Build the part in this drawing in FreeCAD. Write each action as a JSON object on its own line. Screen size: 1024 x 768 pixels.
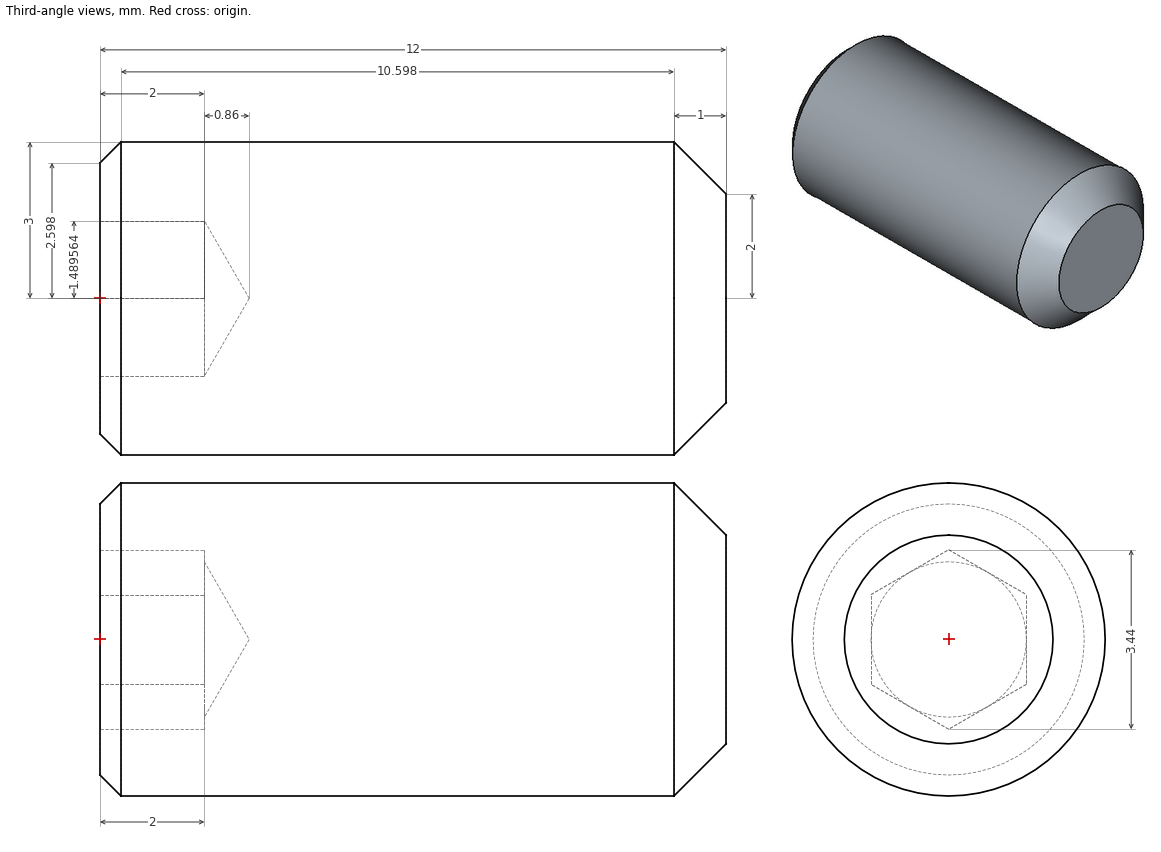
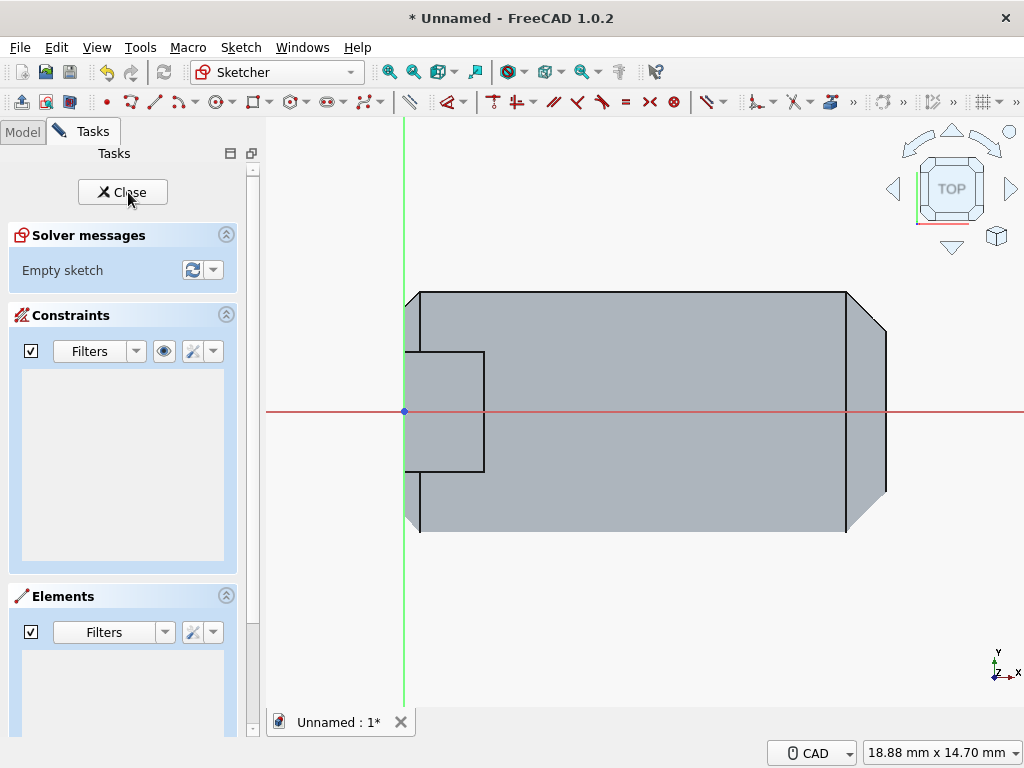
{"action": "scroll", "coordinate": [412, 369], "scroll_direction": "up", "scroll_amount": 6}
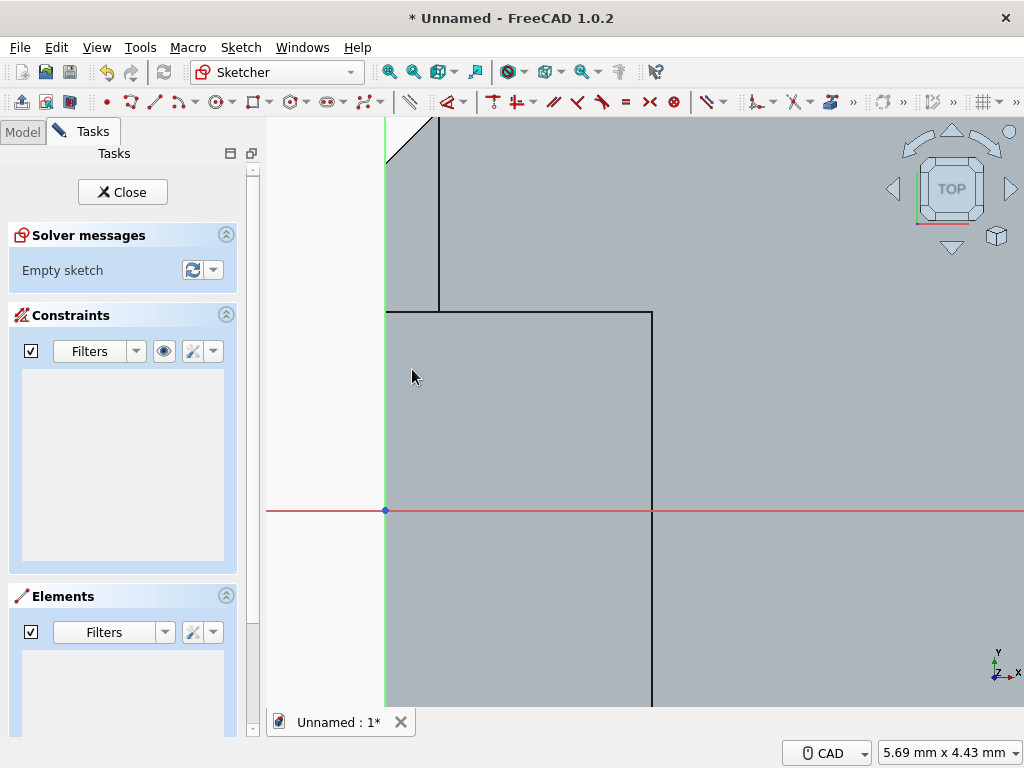
{"action": "key", "text": "g m"}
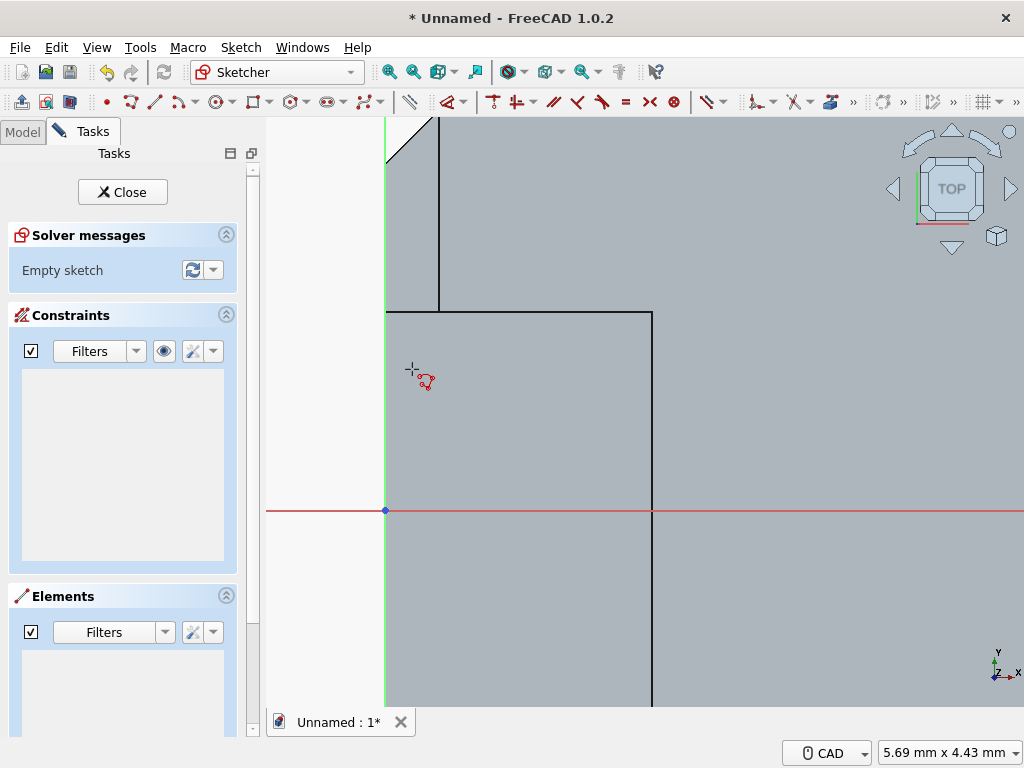
{"action": "left_click", "coordinate": [652, 511]}
{"action": "left_click", "coordinate": [767, 502]}
{"action": "left_click", "coordinate": [652, 312]}
{"action": "left_click", "coordinate": [652, 511]}
{"action": "key", "text": "Escape"}
{"action": "key", "text": "Escape"}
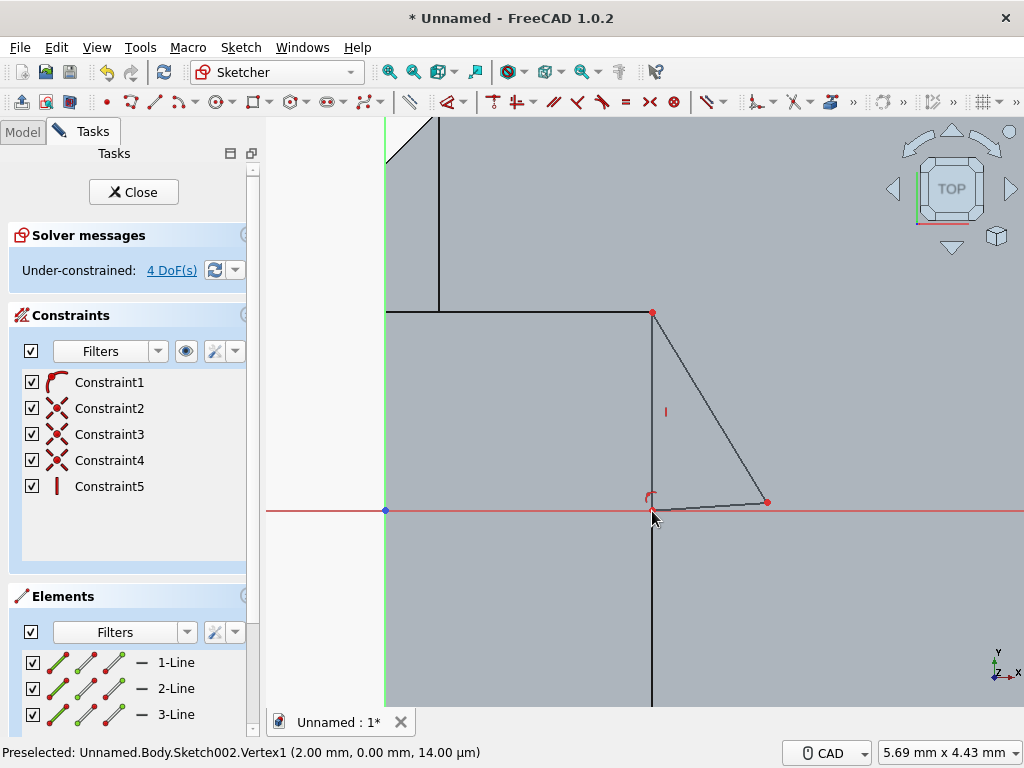
{"action": "left_click", "coordinate": [686, 508]}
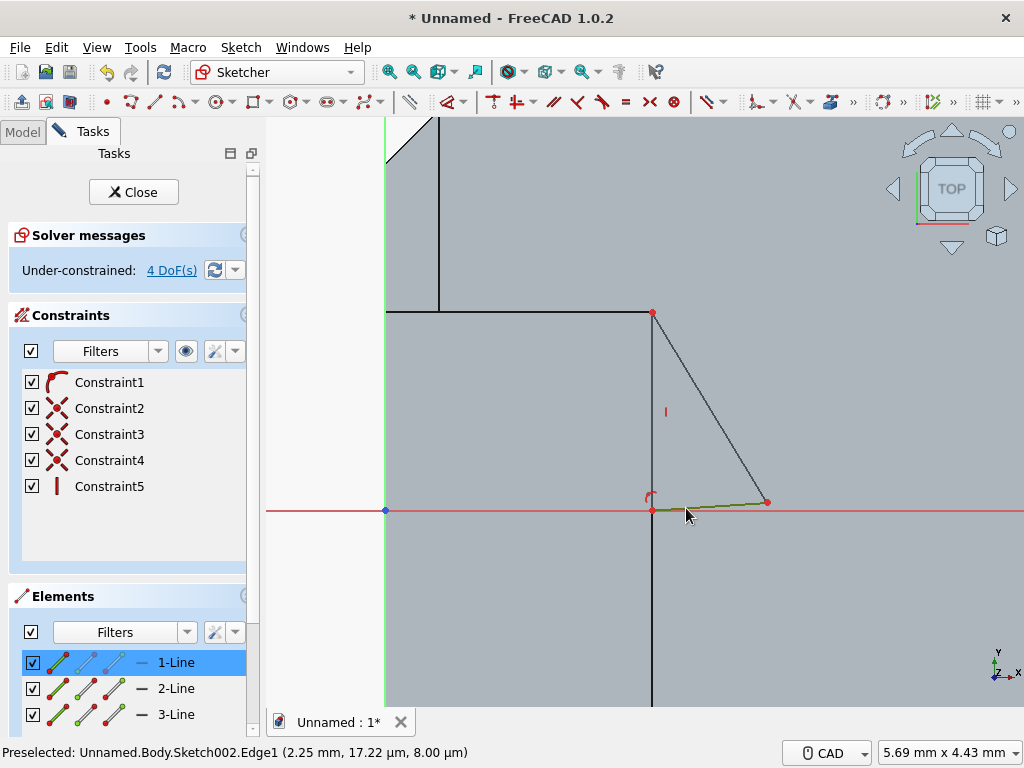
{"action": "key", "text": "h"}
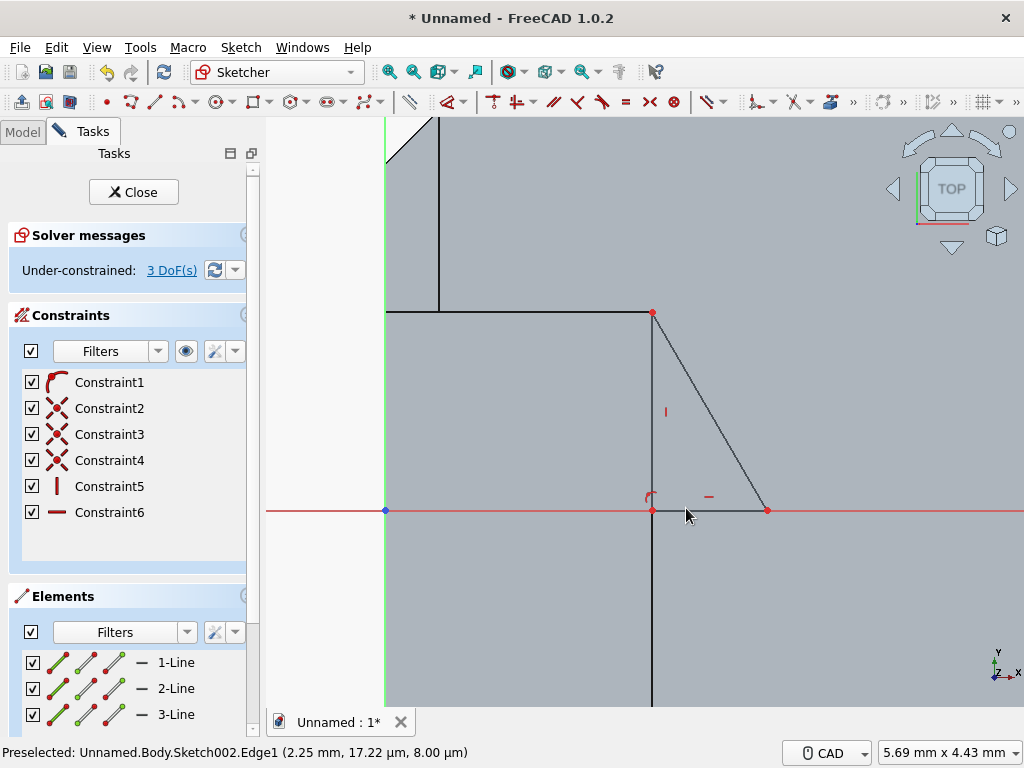
{"action": "left_click", "coordinate": [448, 102]}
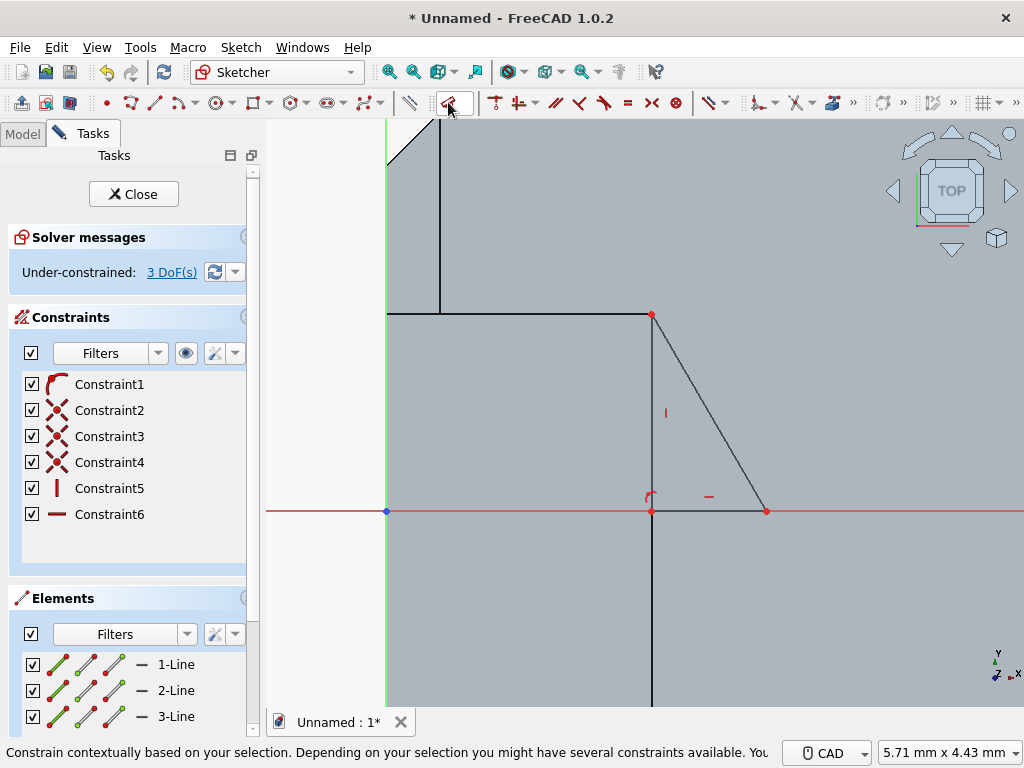
{"action": "left_click", "coordinate": [652, 511]}
{"action": "left_click", "coordinate": [519, 545]}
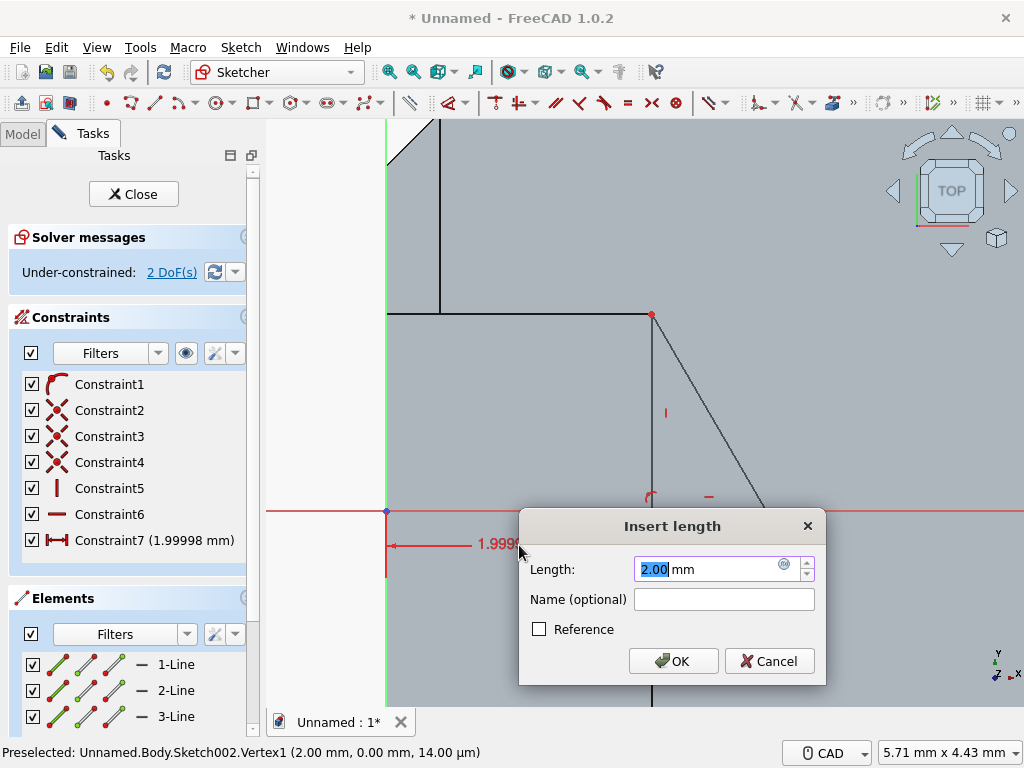
{"action": "type", "text": "2"}
{"action": "key", "text": "Return"}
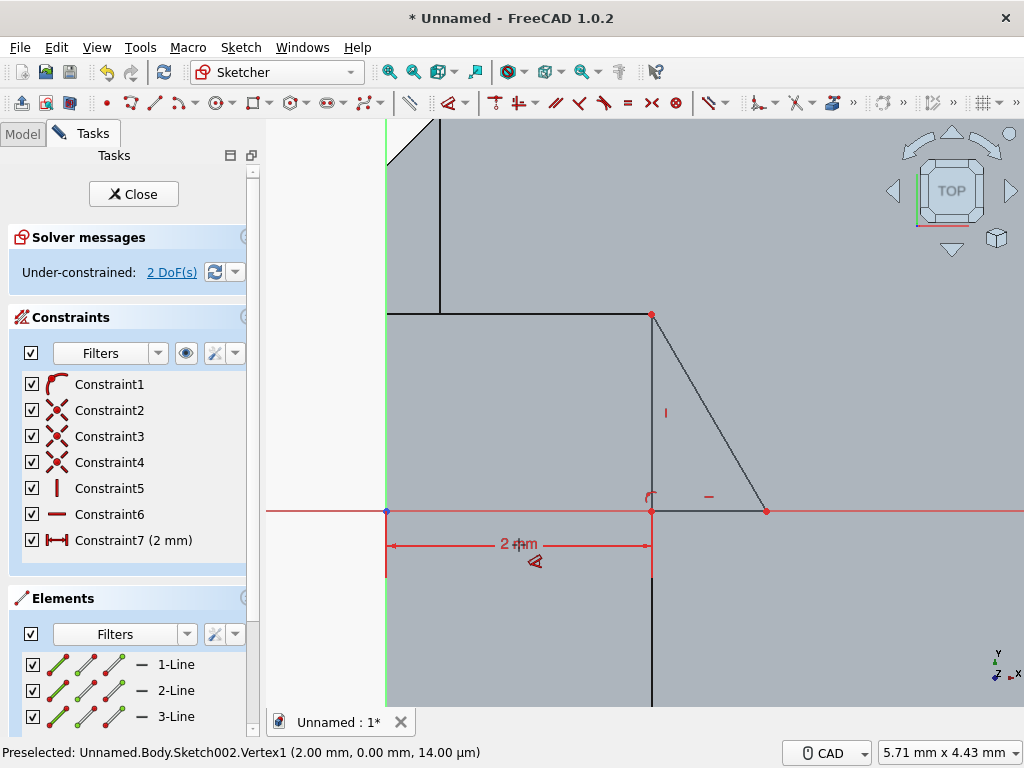
{"action": "left_click", "coordinate": [686, 511]}
{"action": "left_click", "coordinate": [709, 545]}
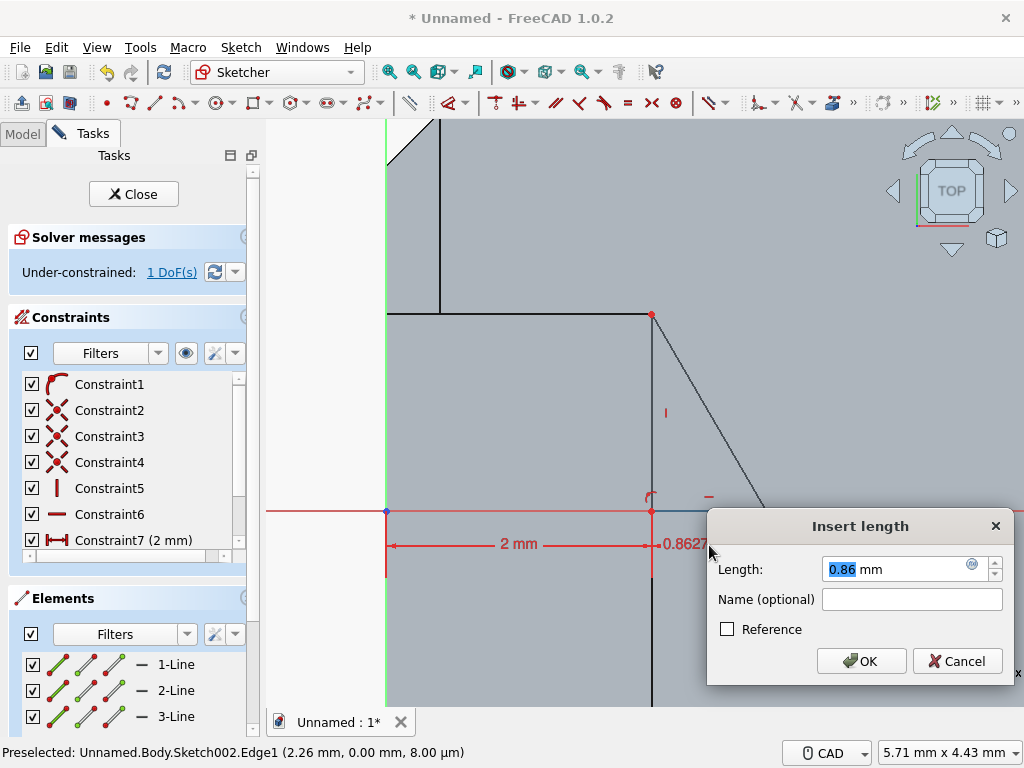
{"action": "type", "text": "0.86"}
{"action": "key", "text": "Return"}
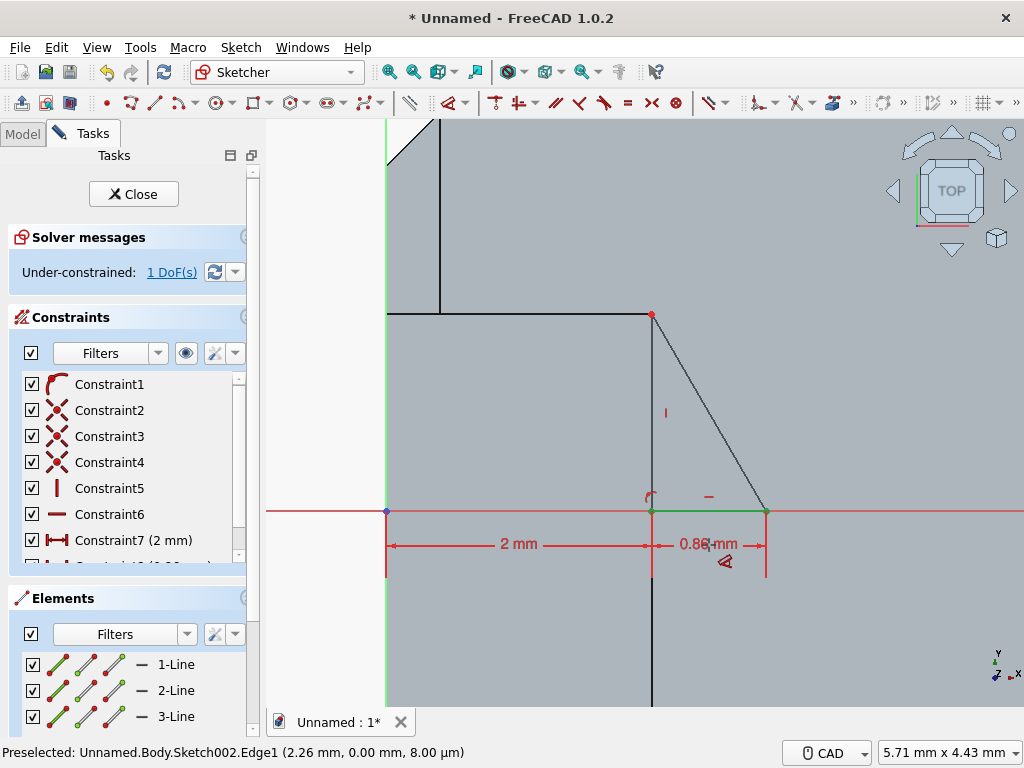
{"action": "left_click", "coordinate": [652, 373]}
{"action": "left_click", "coordinate": [686, 413]}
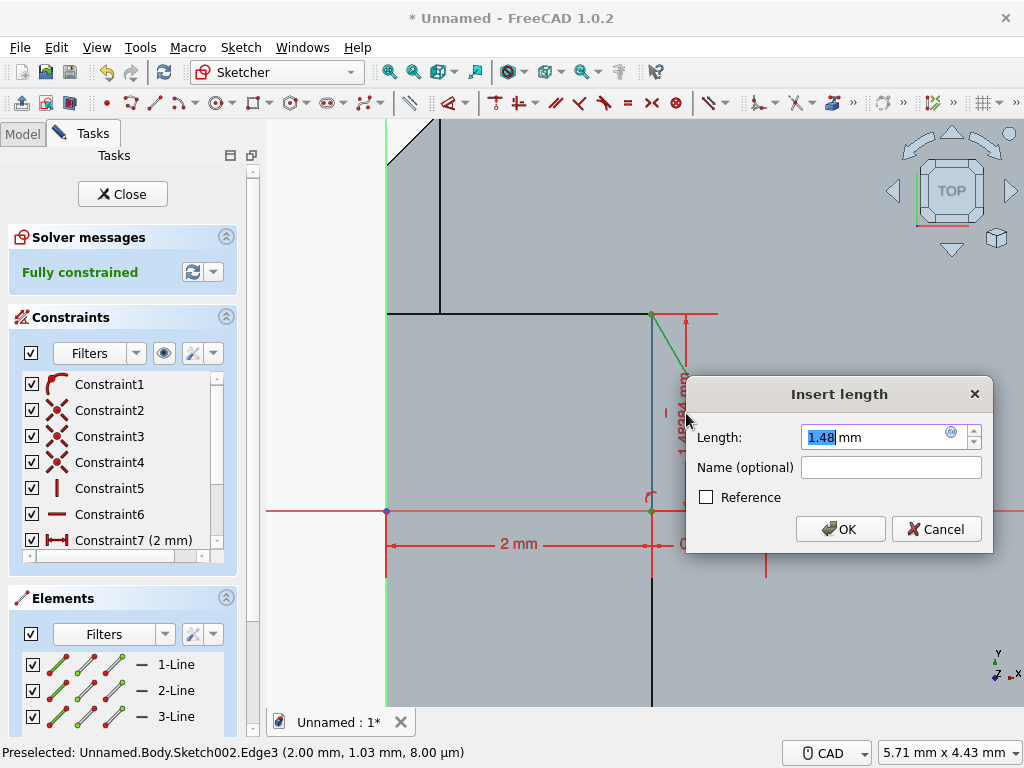
{"action": "type", "text": "1.489564"}
{"action": "key", "text": "Return"}
{"action": "key", "text": "Escape"}